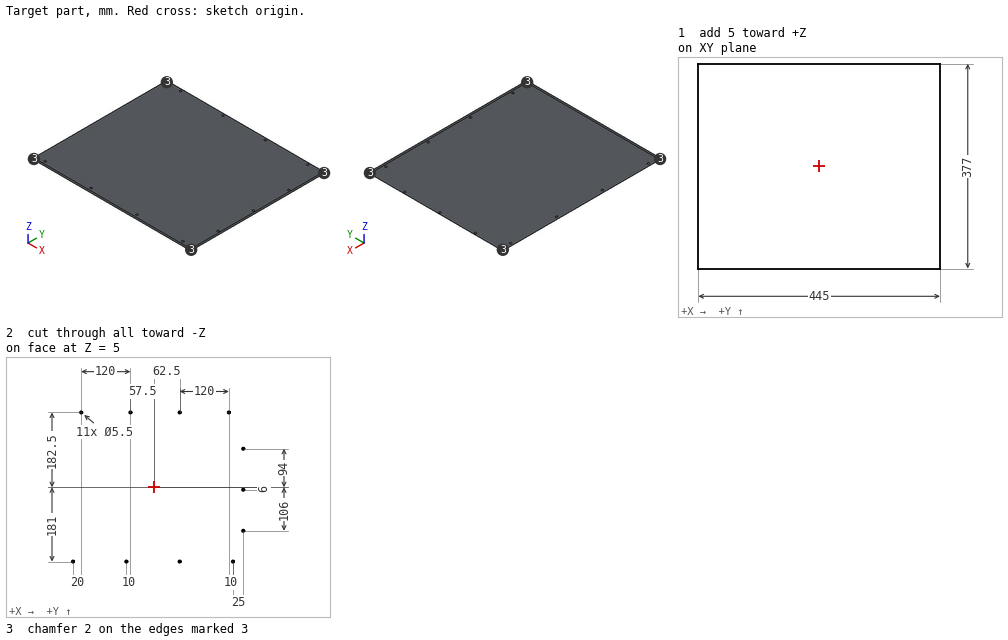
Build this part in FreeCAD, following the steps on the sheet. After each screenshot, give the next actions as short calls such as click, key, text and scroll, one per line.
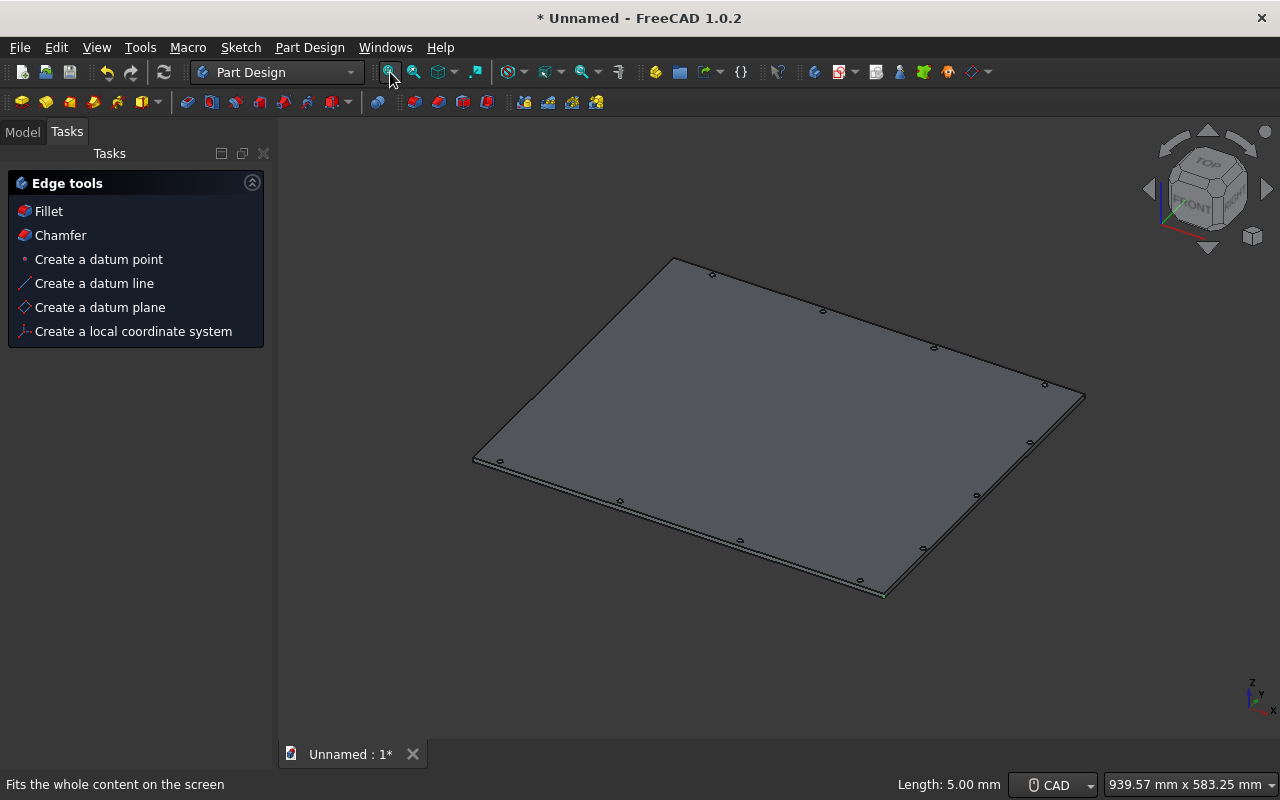
key(0)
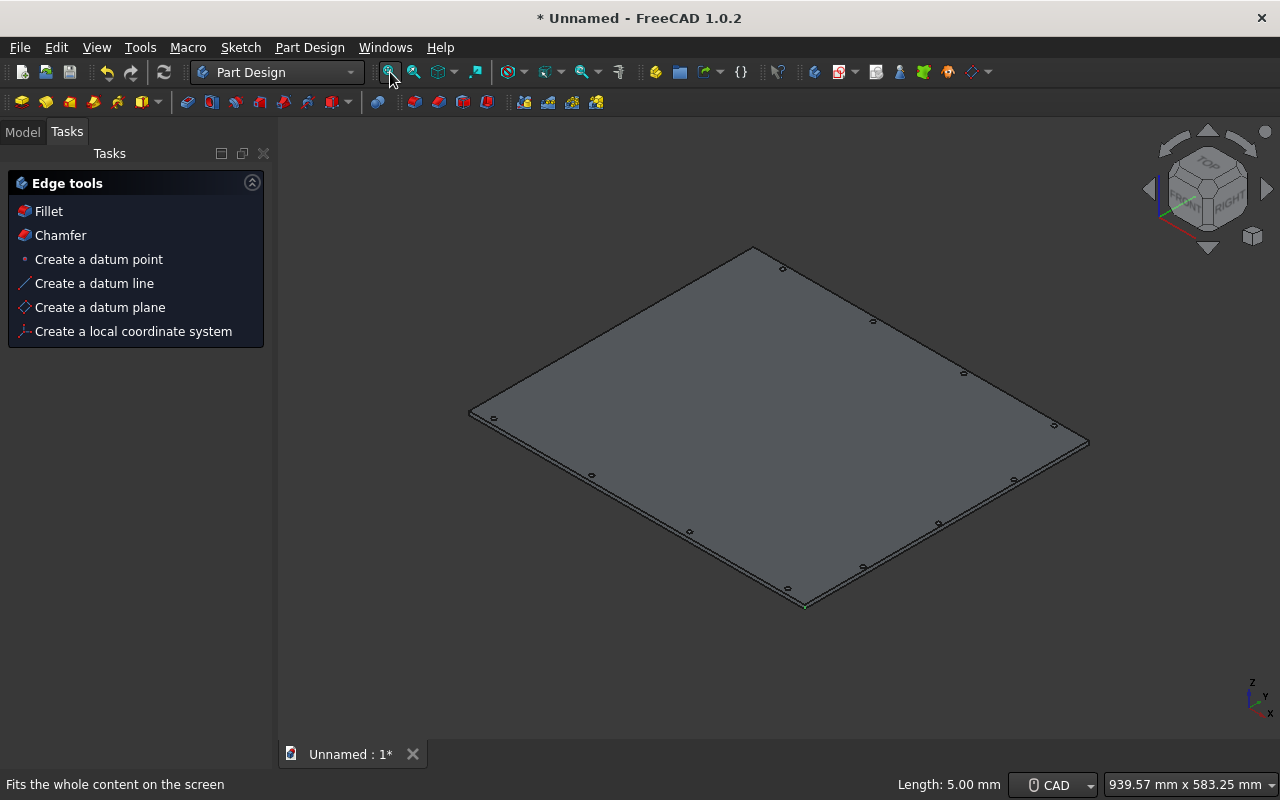
scroll(469, 412, up, 11)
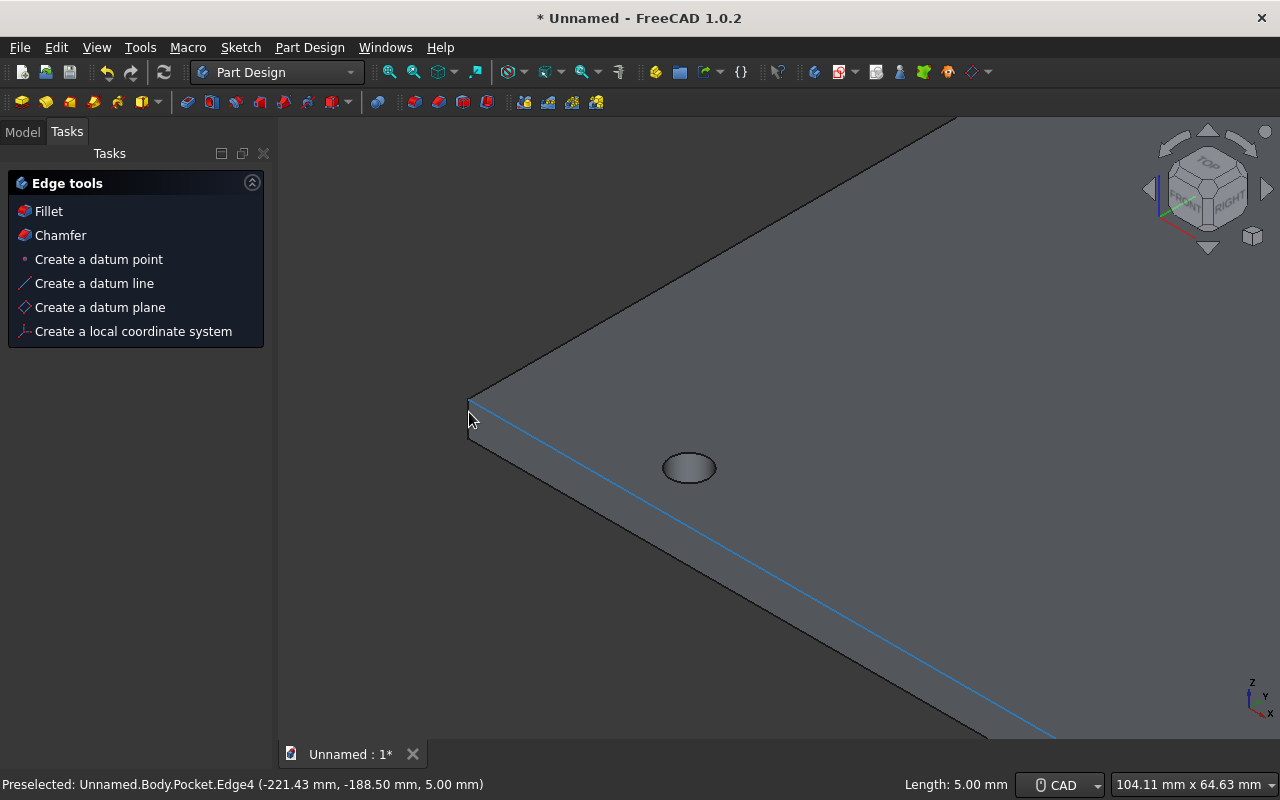
click(390, 72)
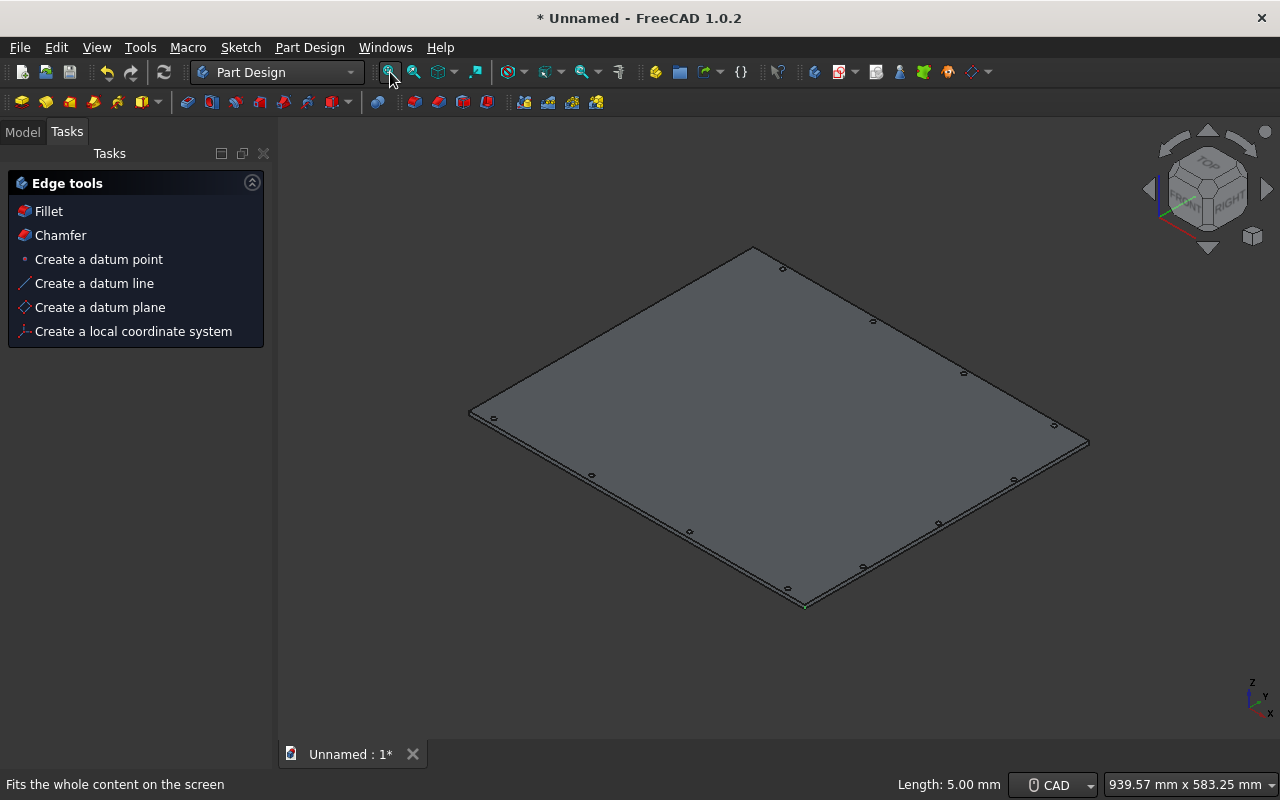
key(2)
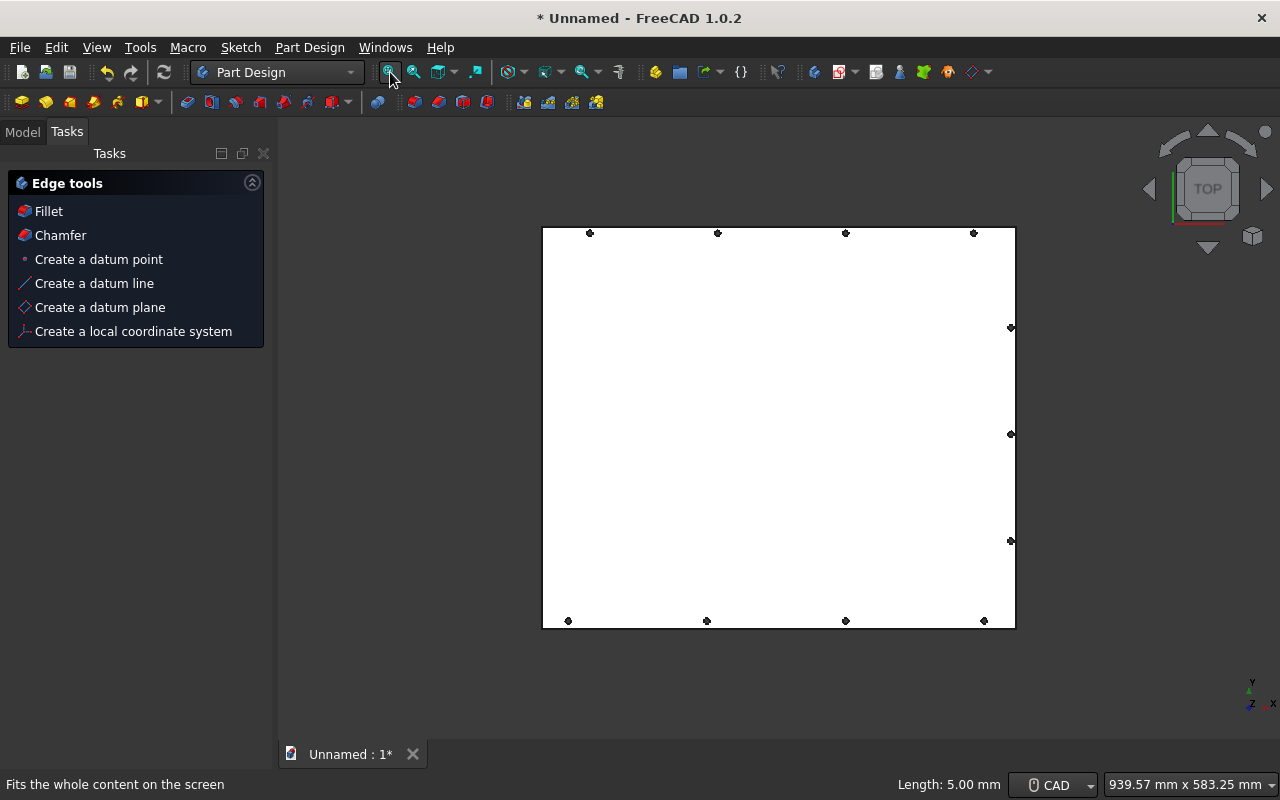
scroll(542, 628, up, 11)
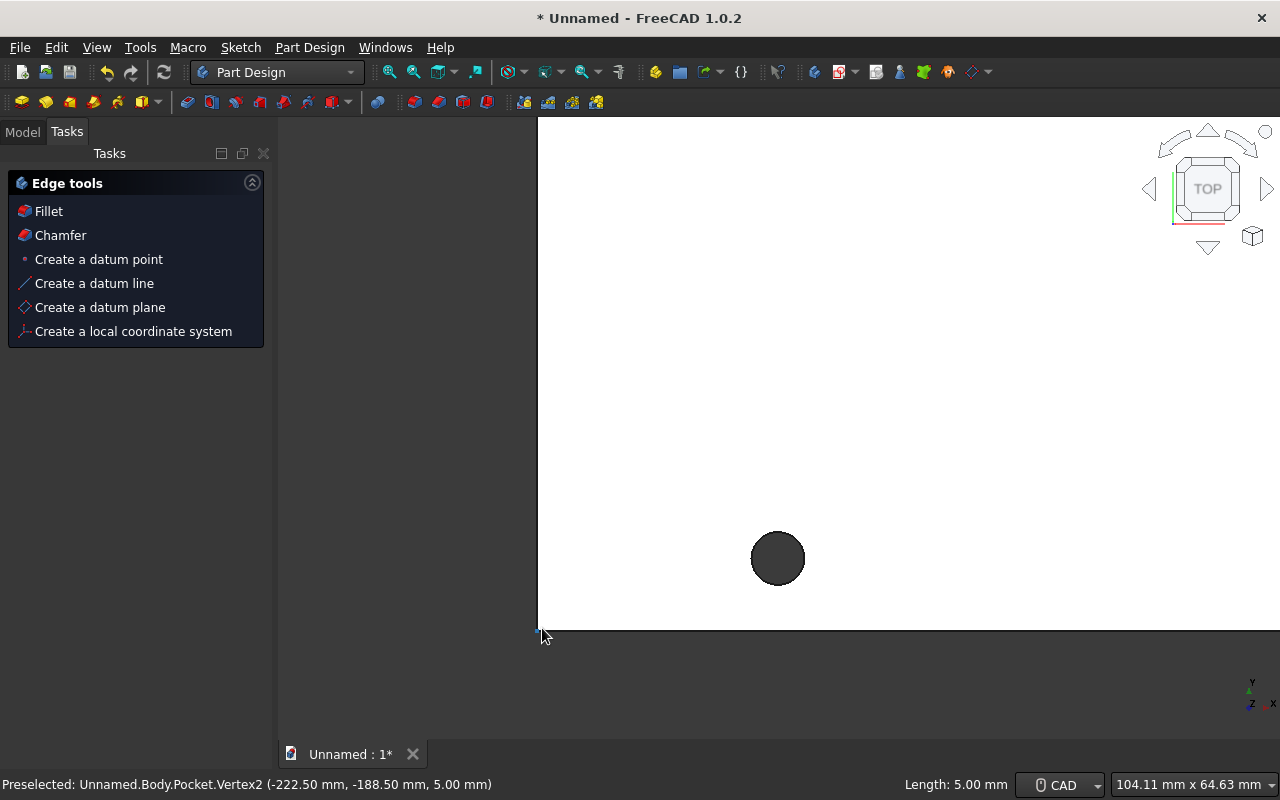
click(390, 72)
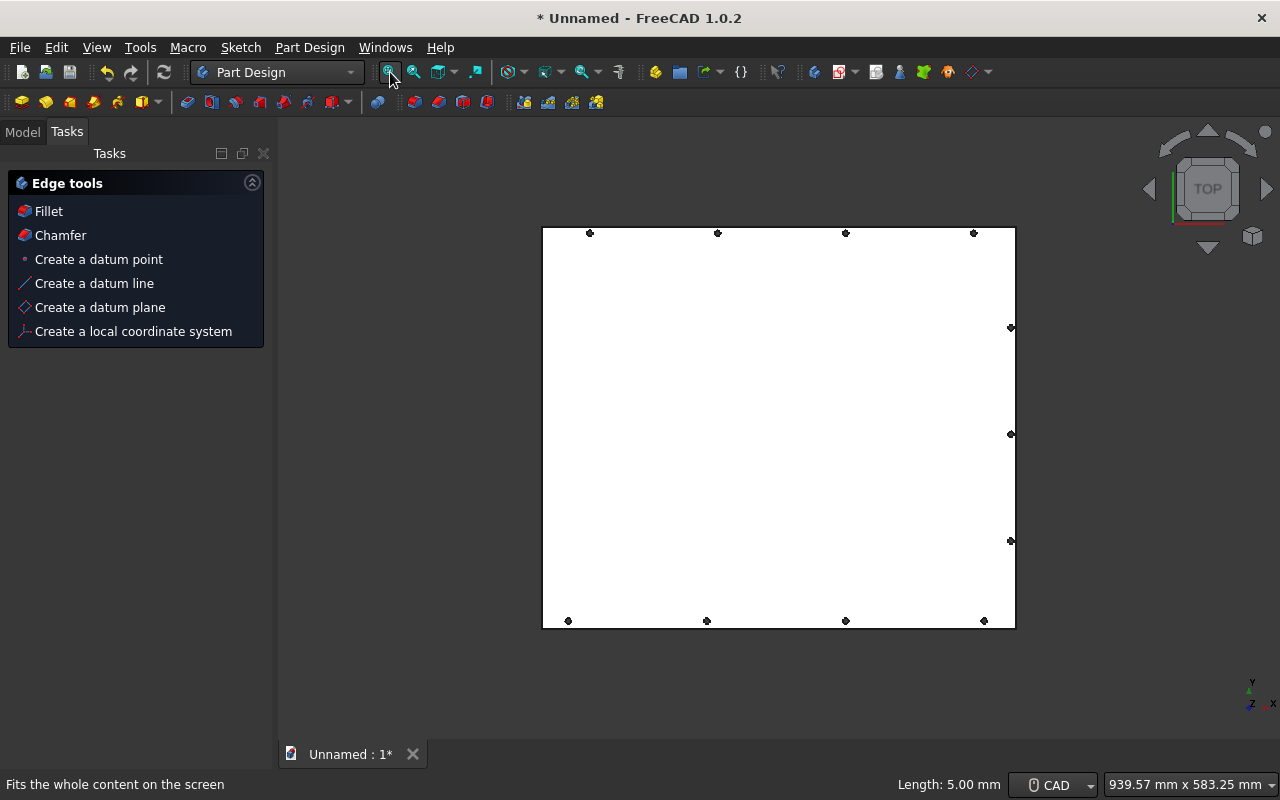
key(1)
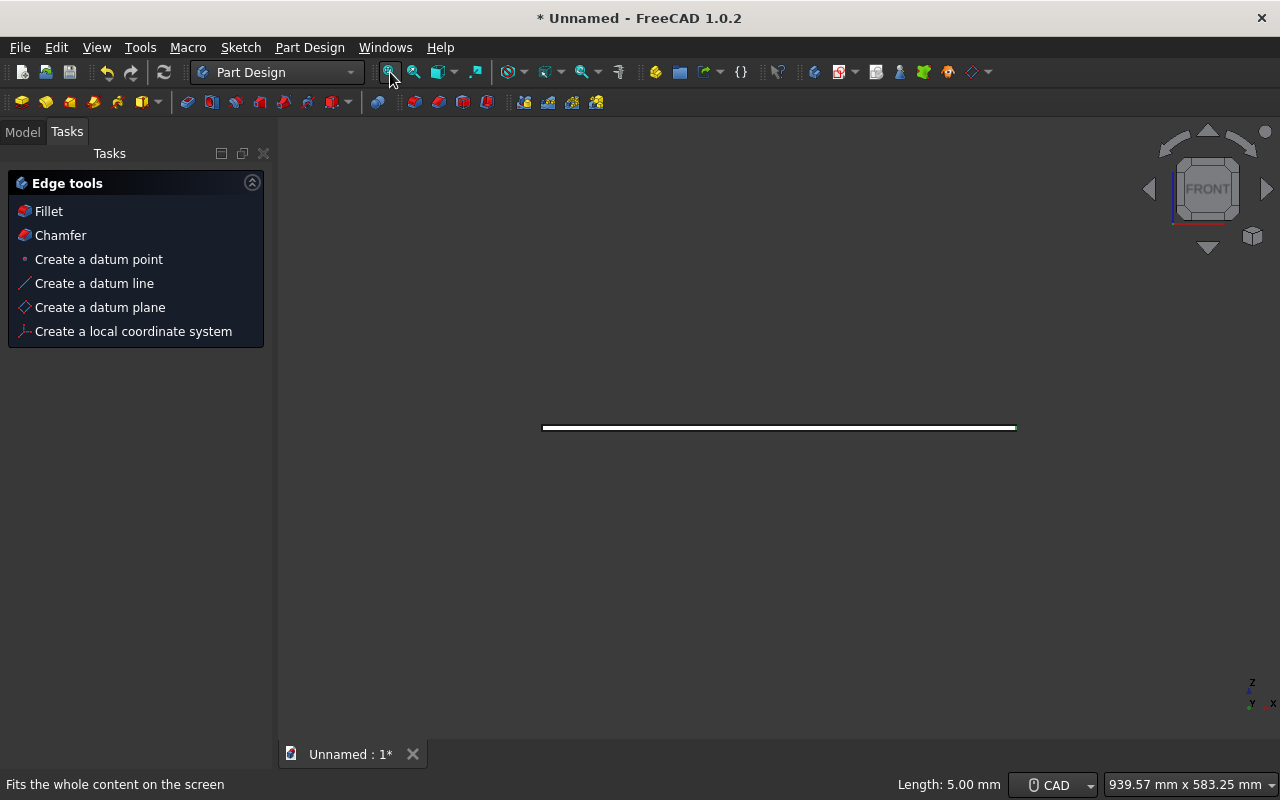
scroll(542, 427, up, 11)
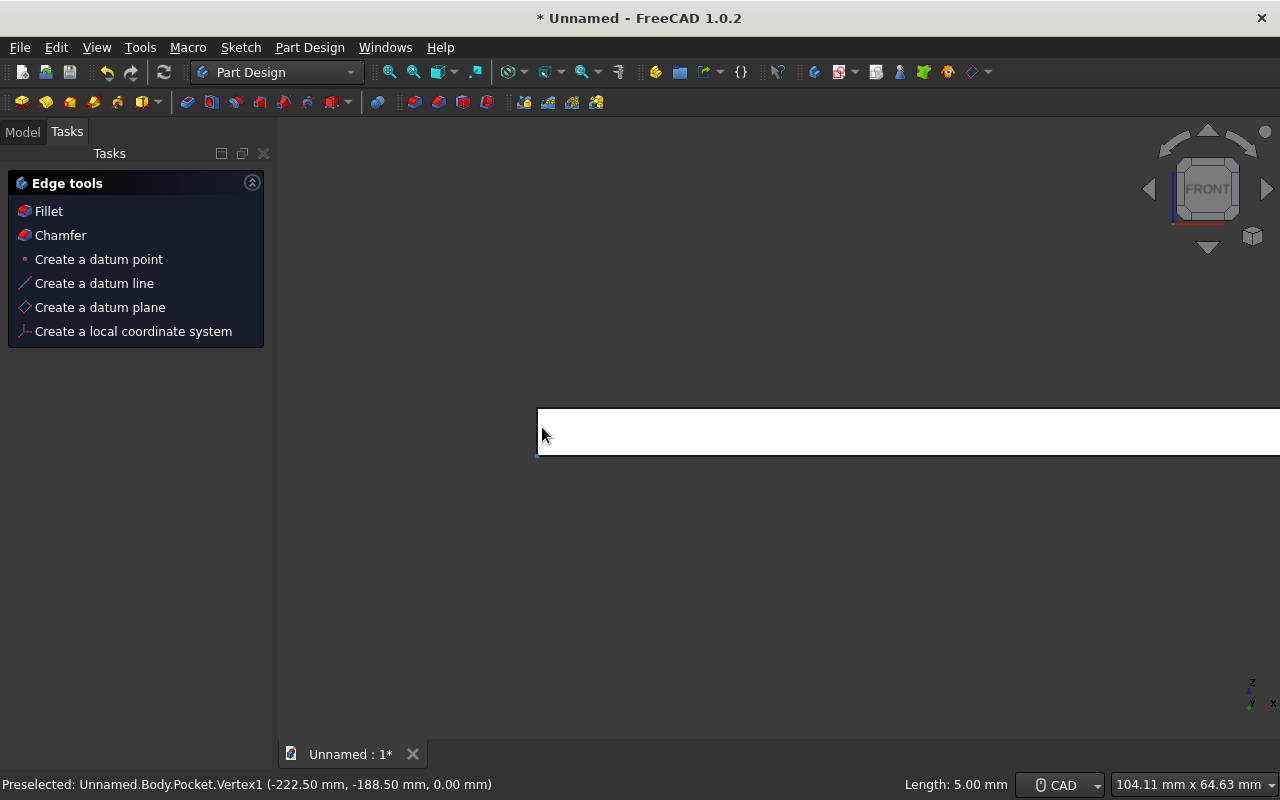
click(537, 431, ctrl)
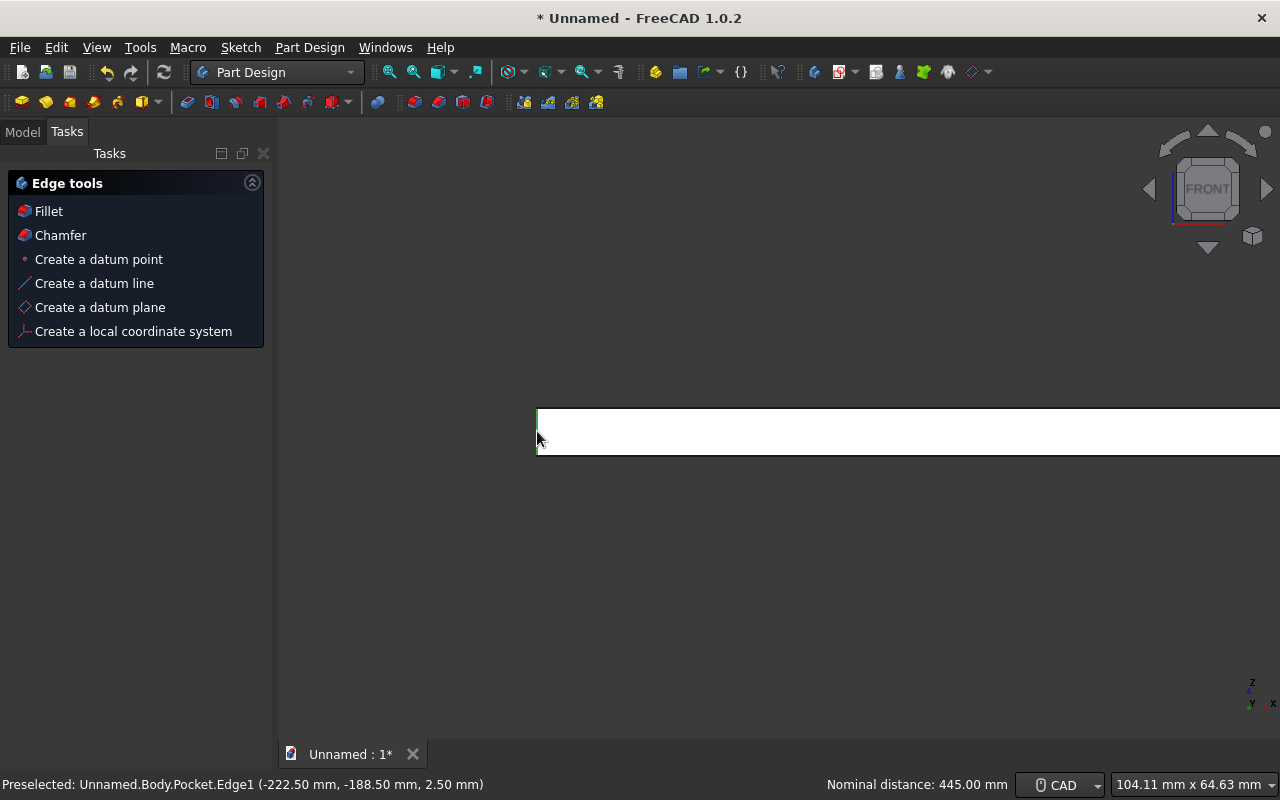
click(390, 72)